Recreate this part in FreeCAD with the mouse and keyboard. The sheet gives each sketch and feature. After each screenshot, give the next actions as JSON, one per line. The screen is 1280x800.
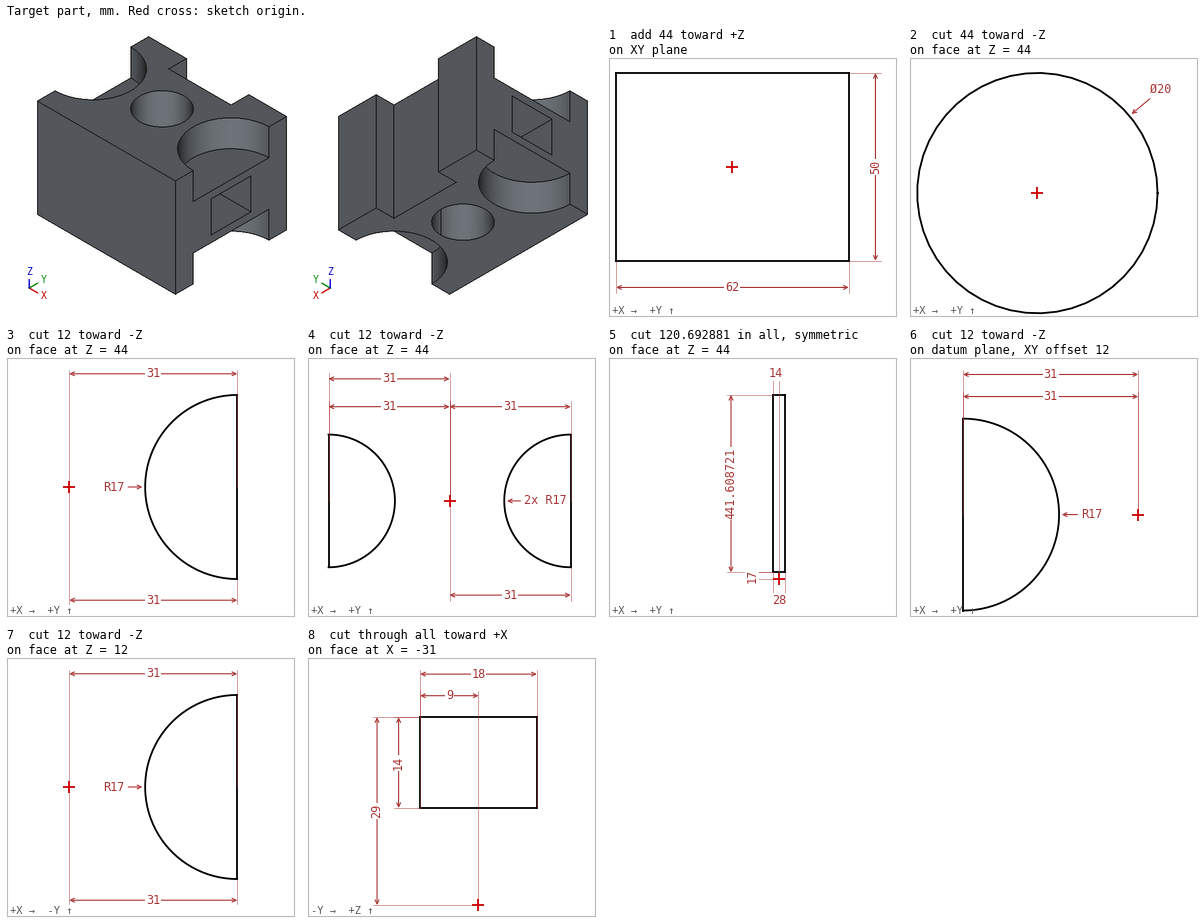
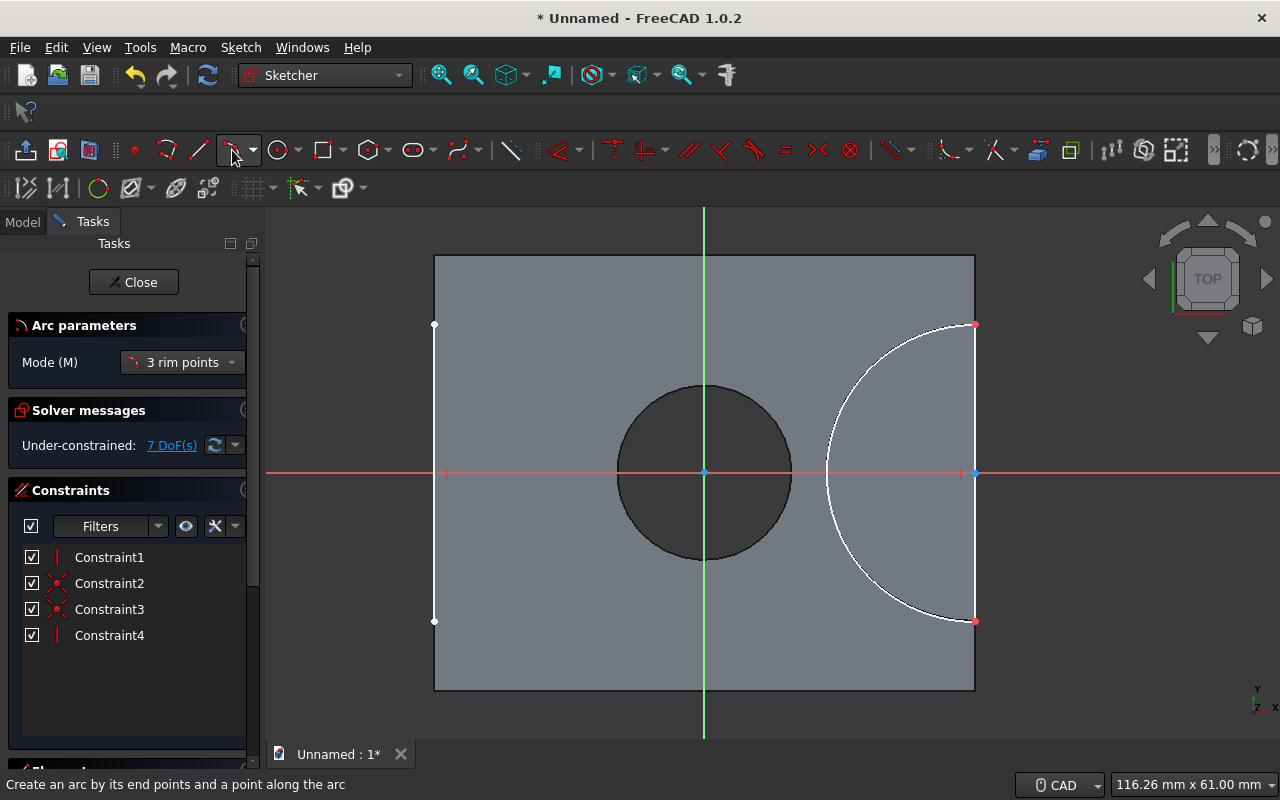
{"action": "left_click", "coordinate": [434, 622]}
{"action": "left_click", "coordinate": [434, 325]}
{"action": "left_click", "coordinate": [575, 519]}
{"action": "key", "text": "Escape"}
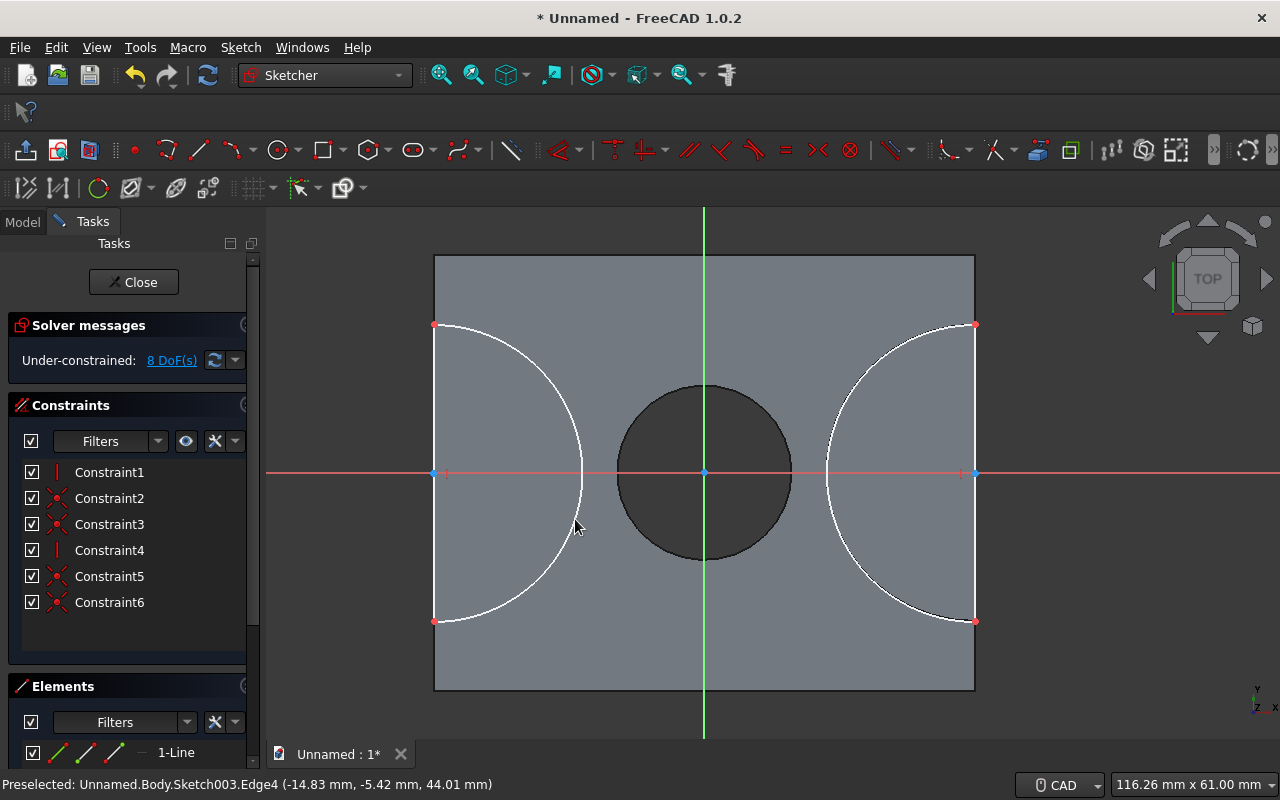
{"action": "left_click", "coordinate": [855, 386]}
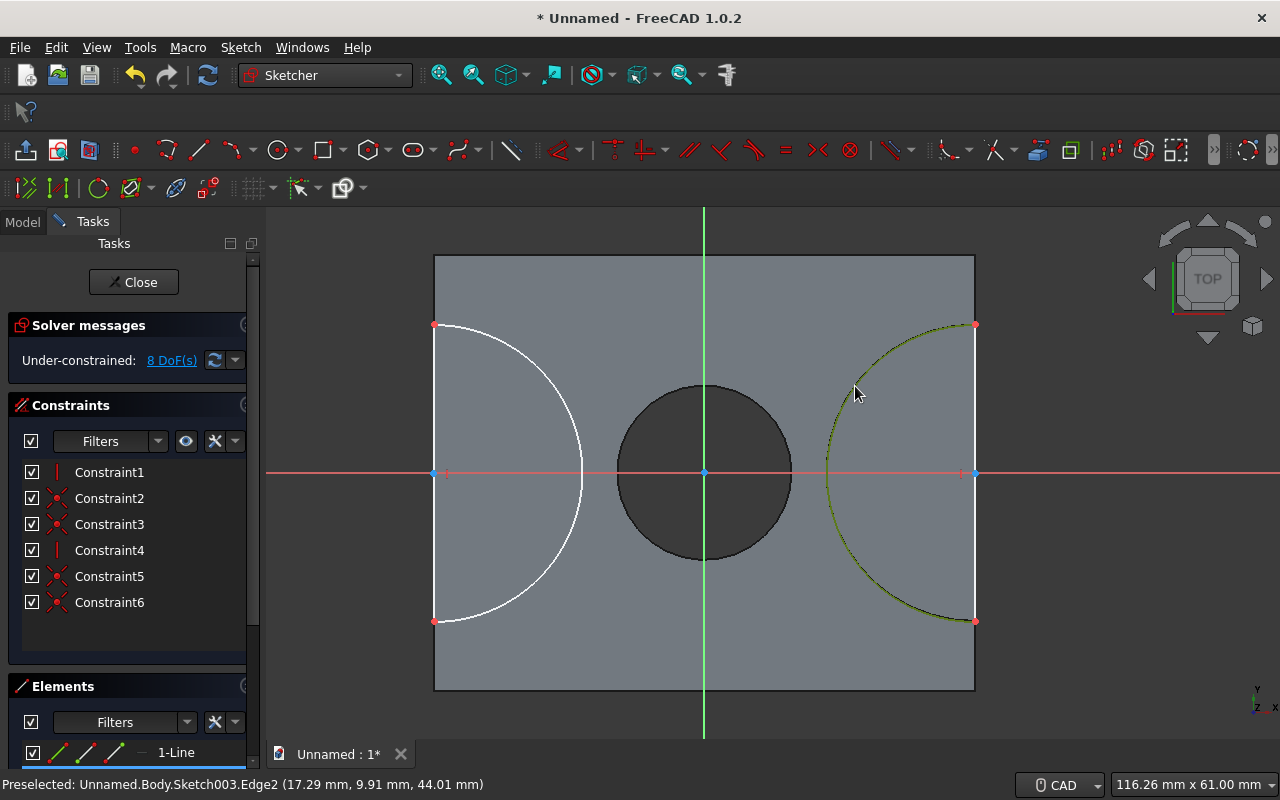
{"action": "left_click", "coordinate": [554, 561]}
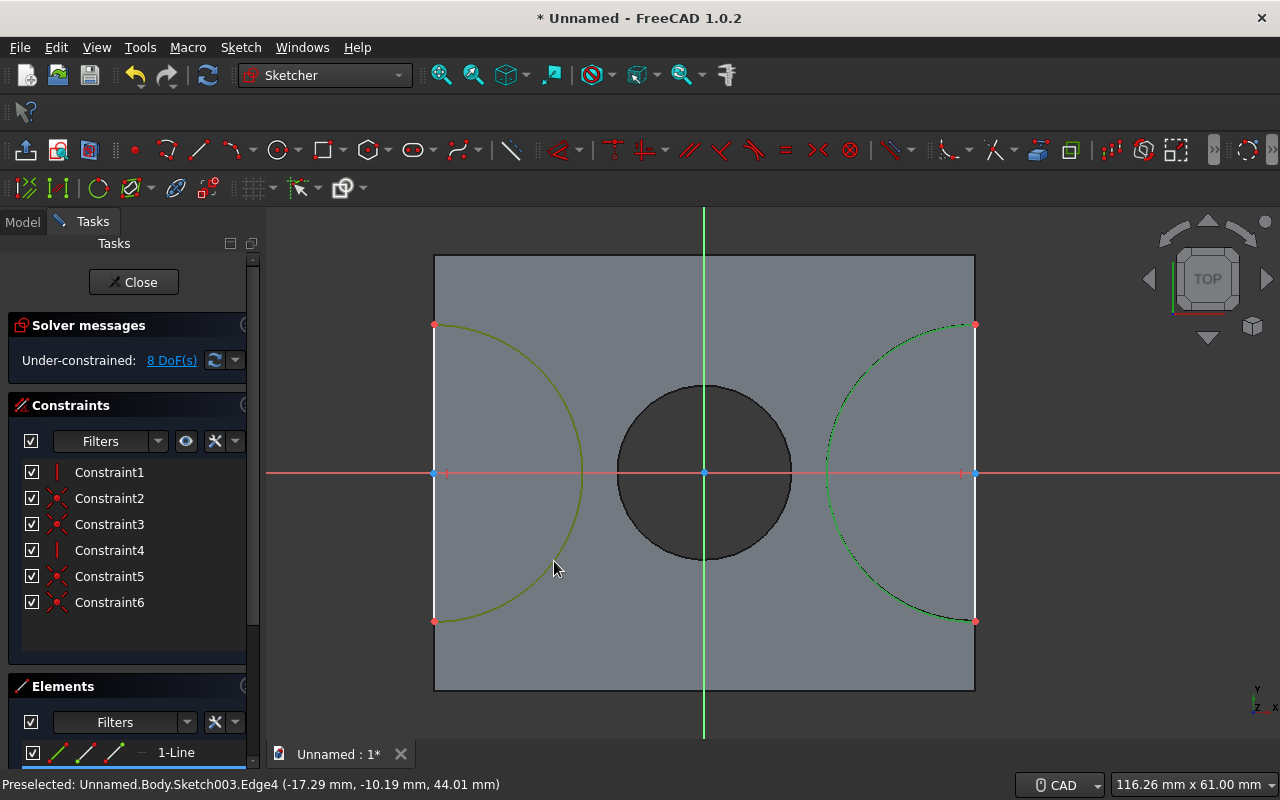
{"action": "key", "text": "e"}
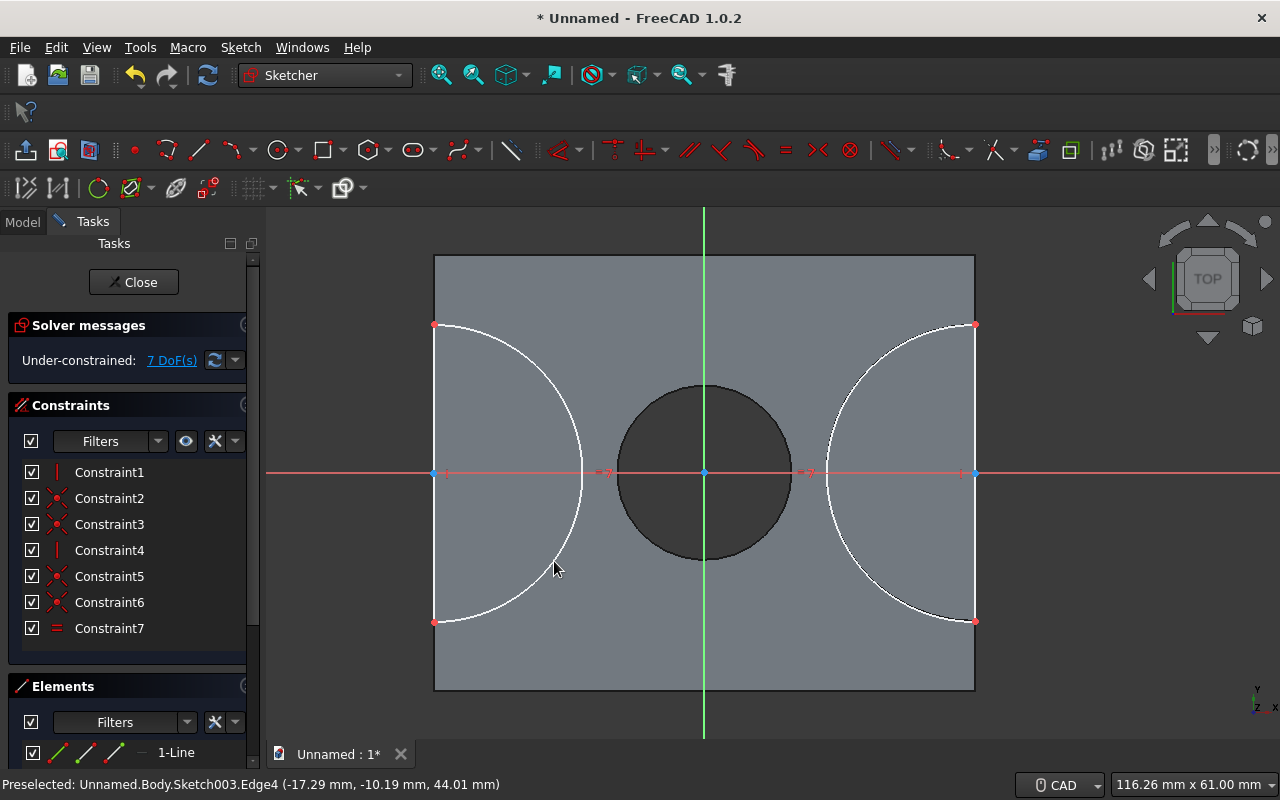
{"action": "left_click", "coordinate": [975, 474]}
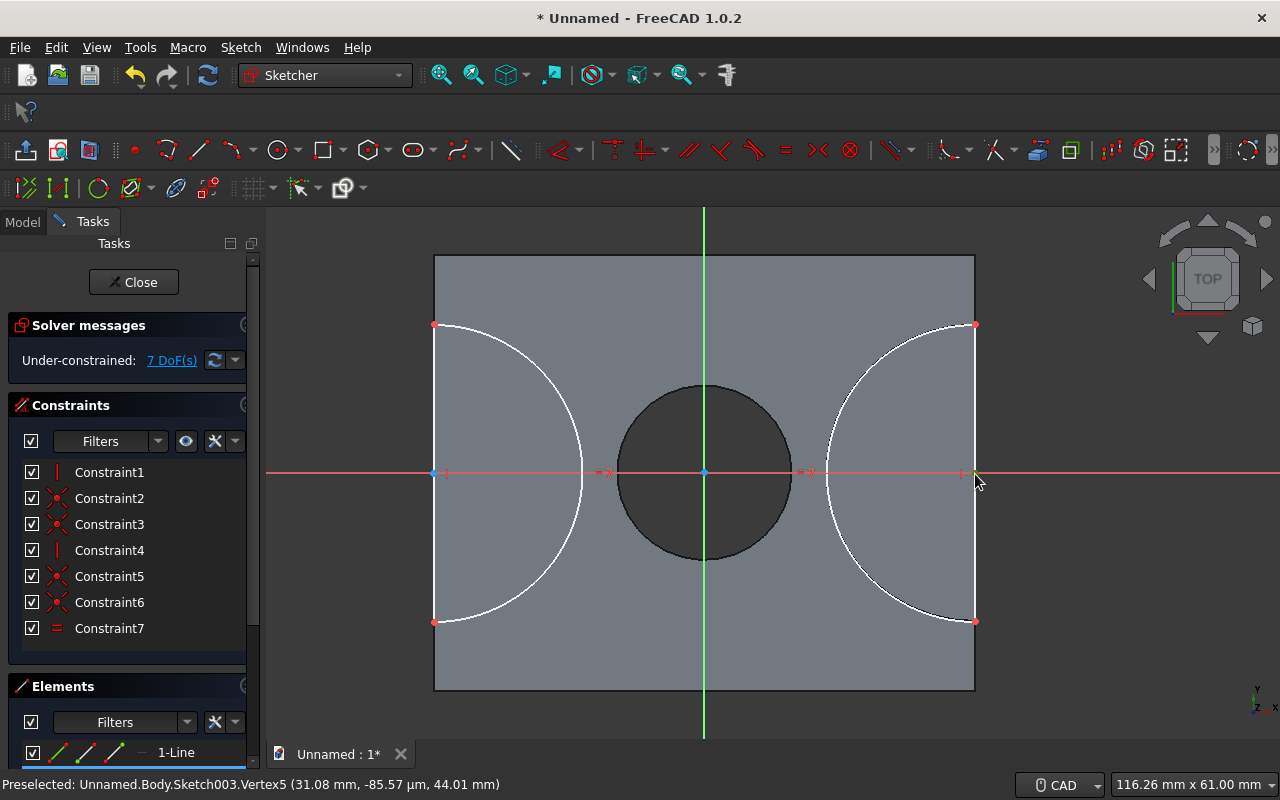
{"action": "left_click", "coordinate": [353, 473]}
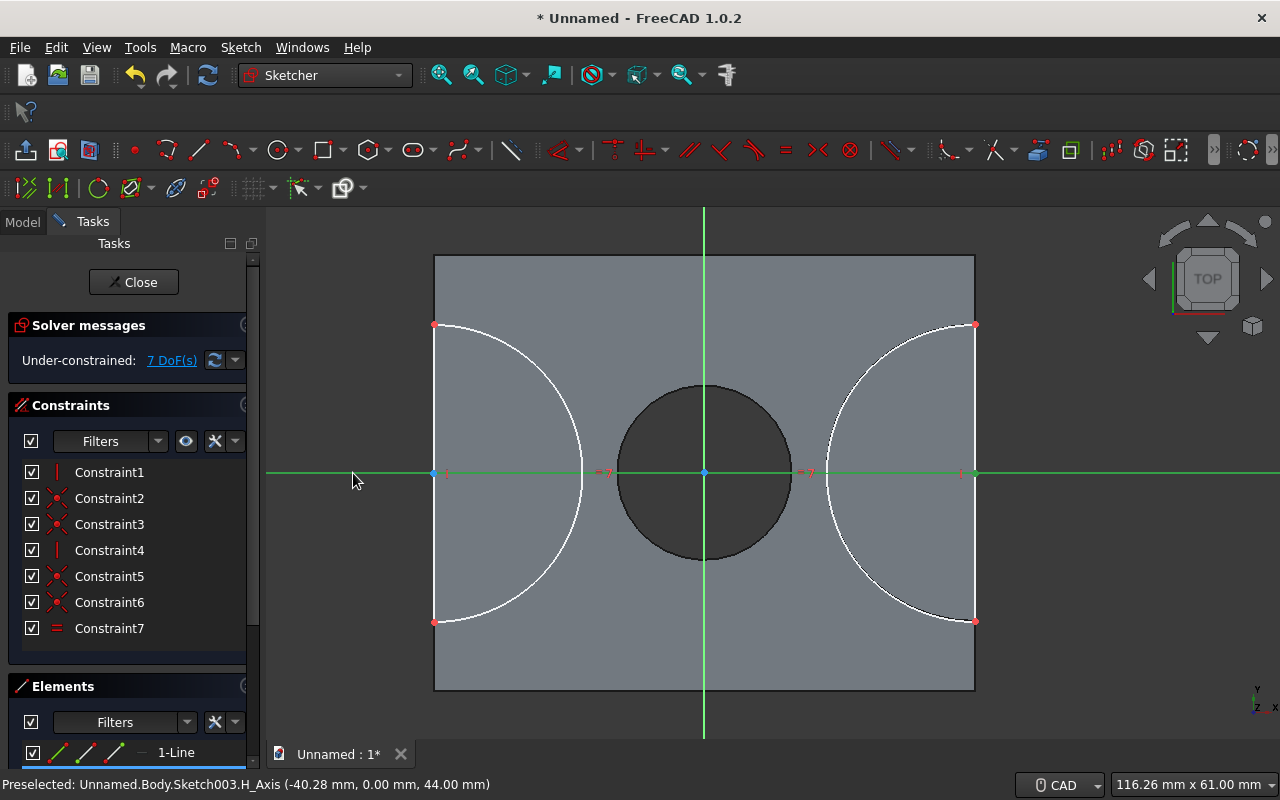
{"action": "key", "text": "c"}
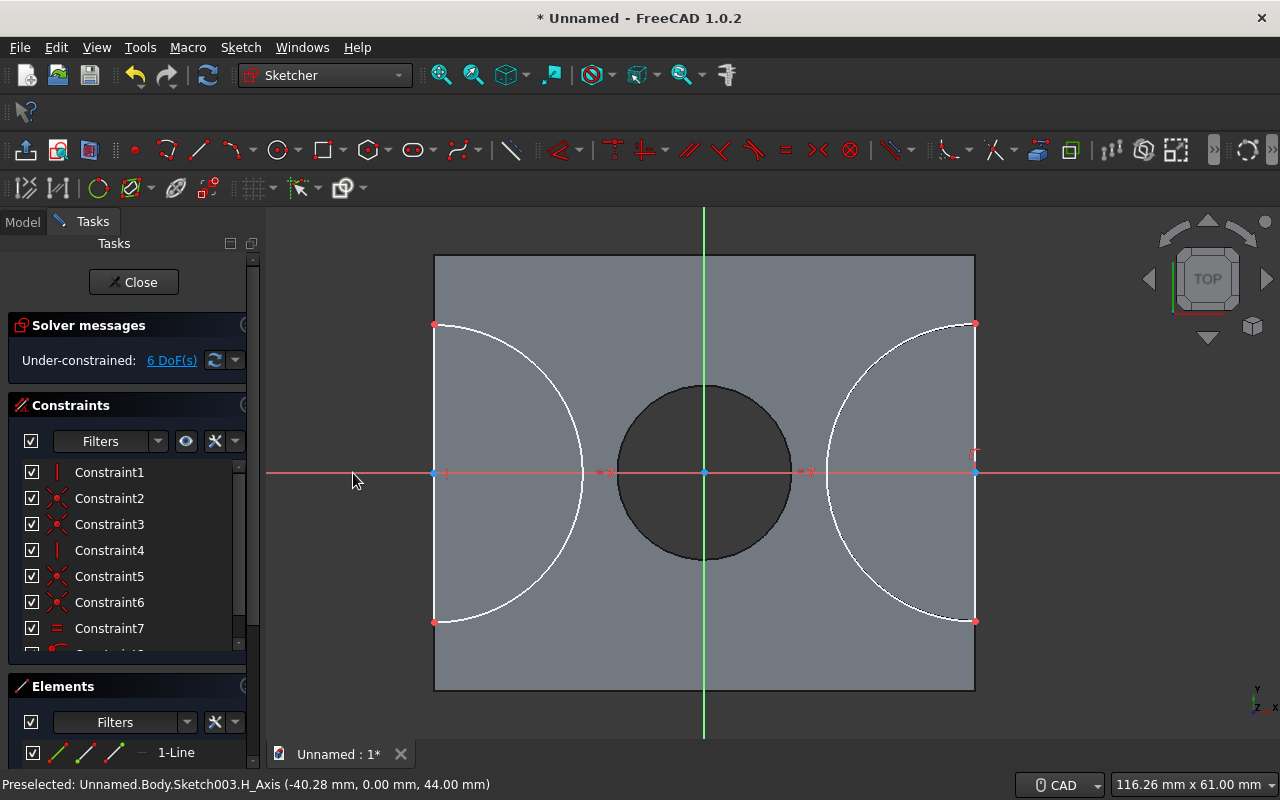
{"action": "left_click", "coordinate": [434, 474]}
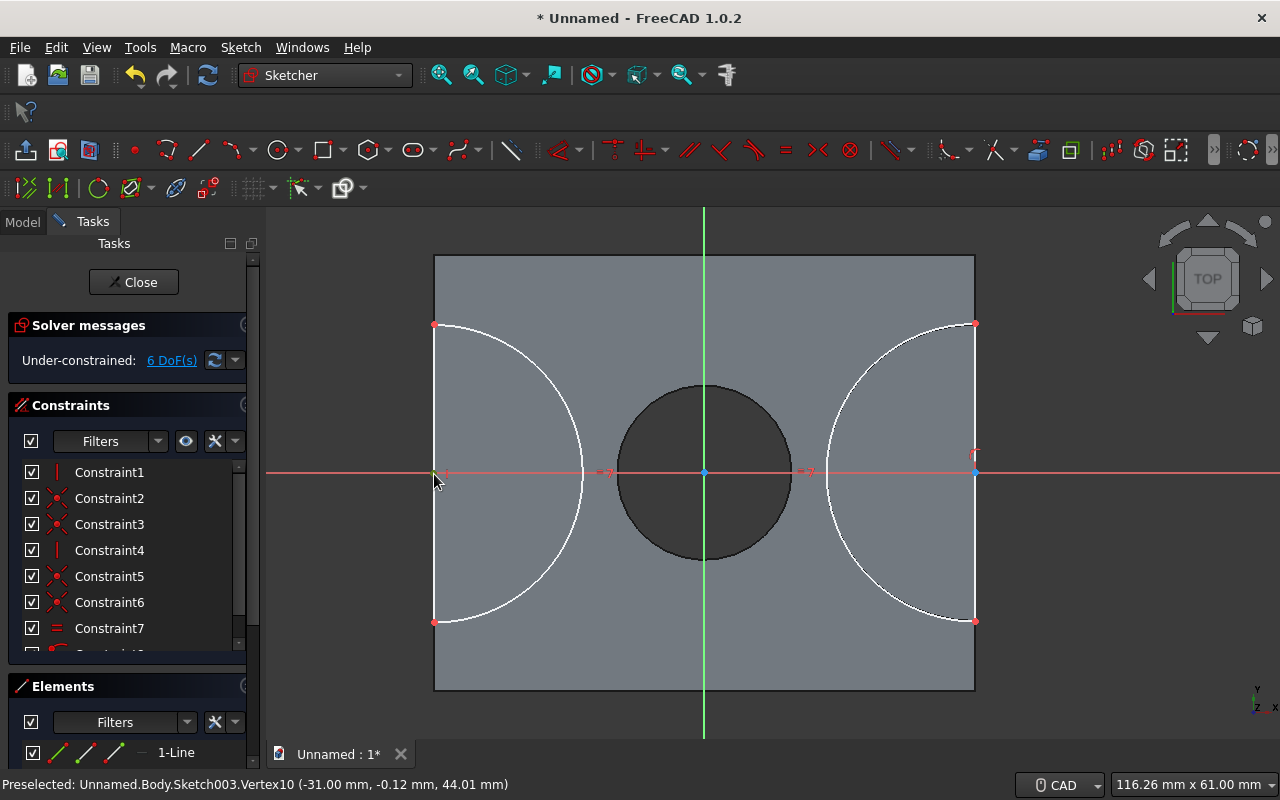
{"action": "left_click", "coordinate": [353, 473]}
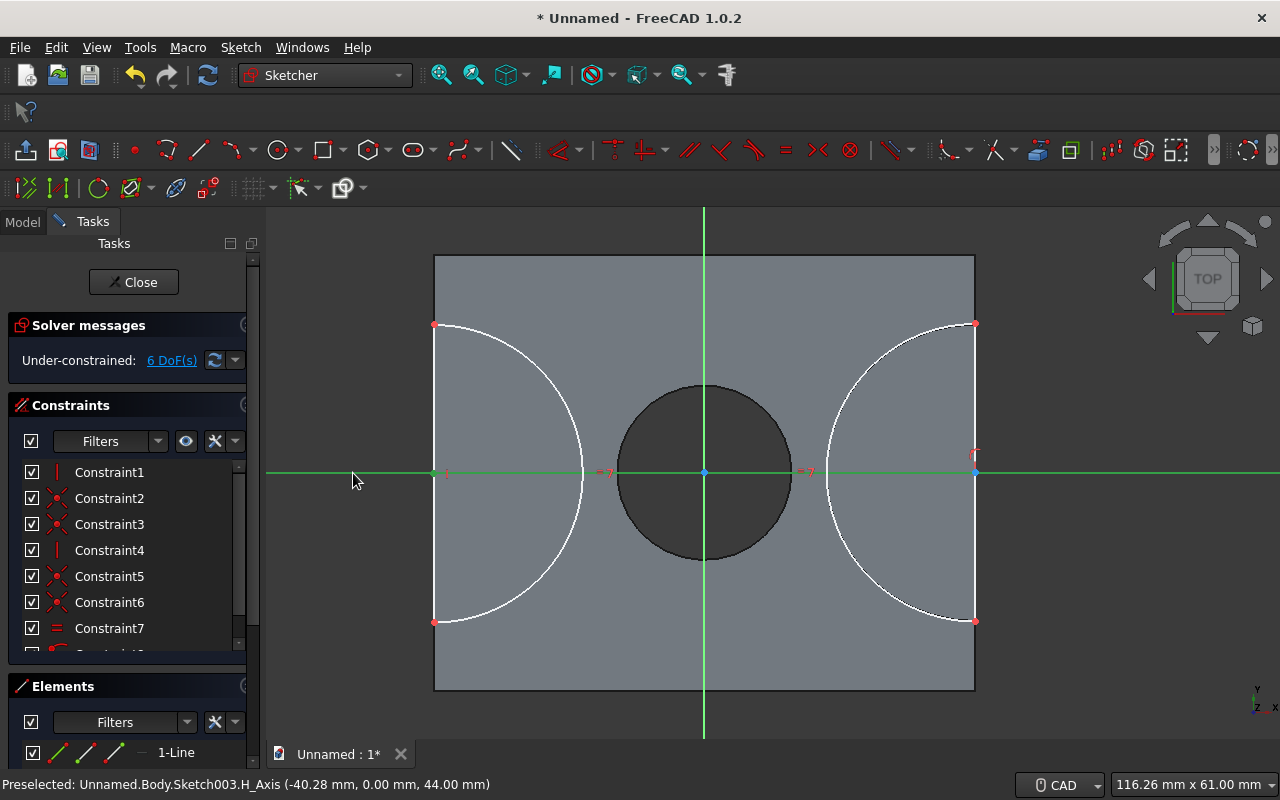
{"action": "key", "text": "c"}